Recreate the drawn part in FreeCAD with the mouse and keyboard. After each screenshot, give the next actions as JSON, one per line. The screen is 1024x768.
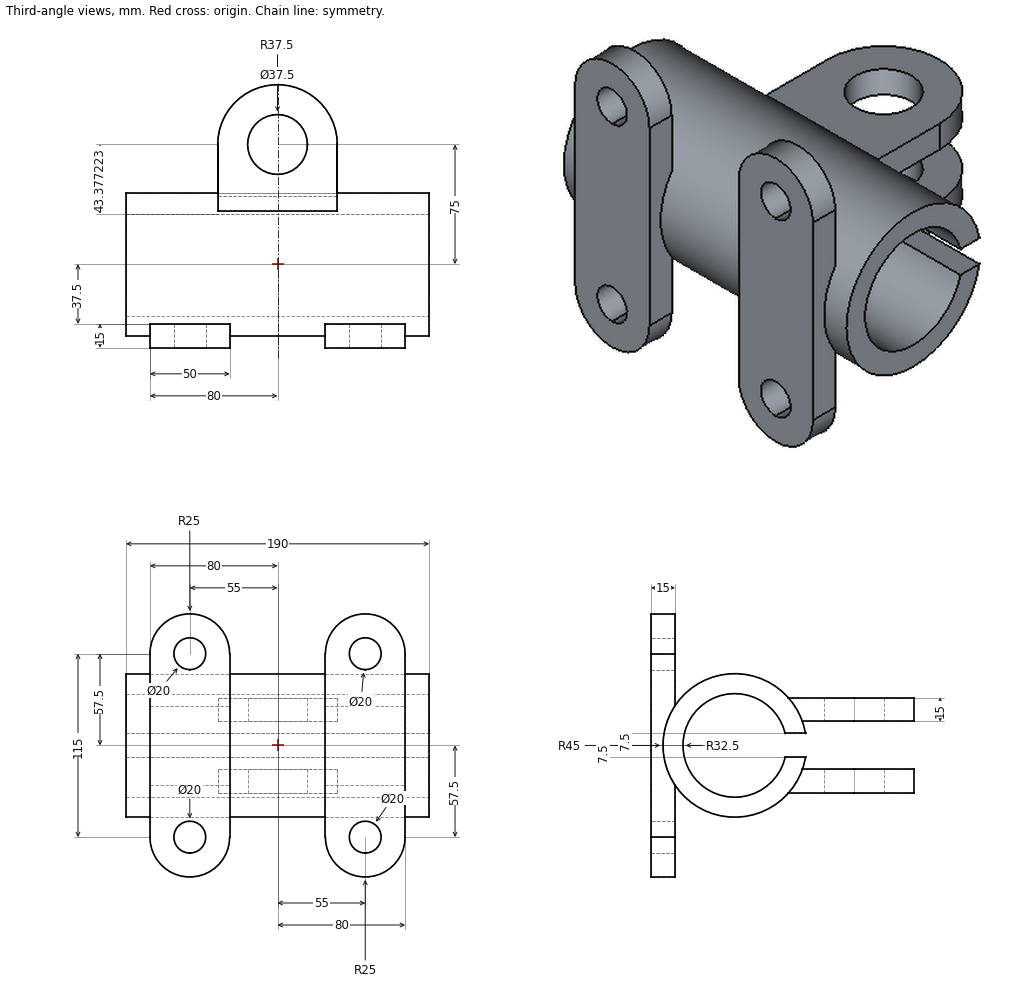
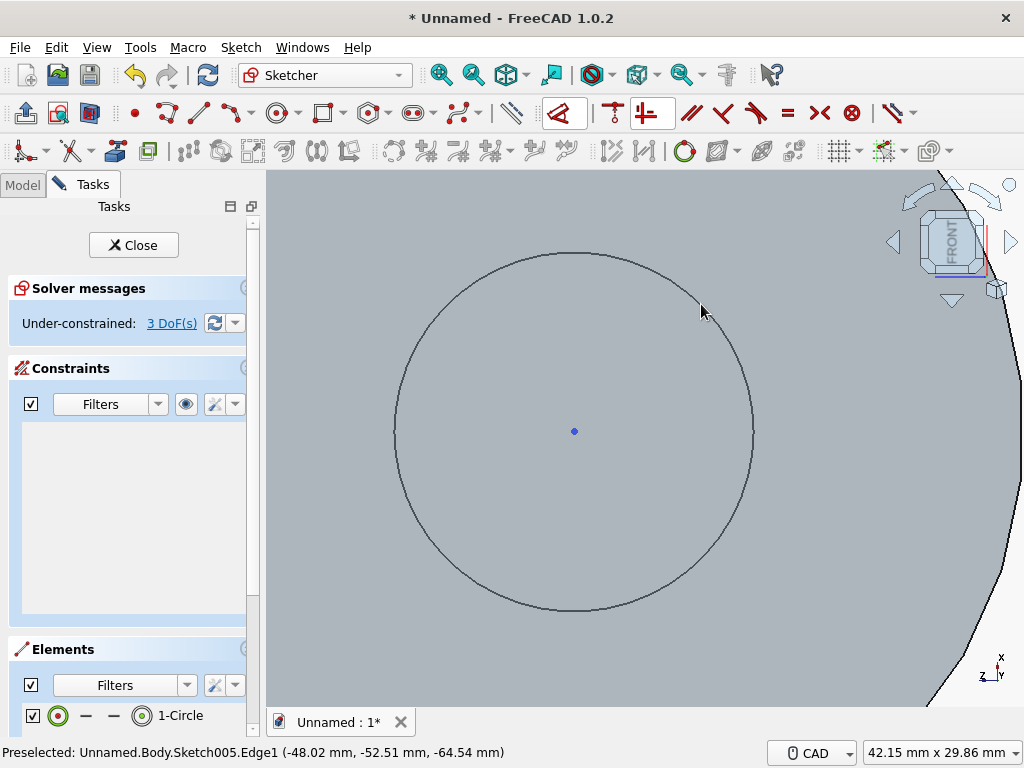
{"action": "left_click", "coordinate": [701, 305]}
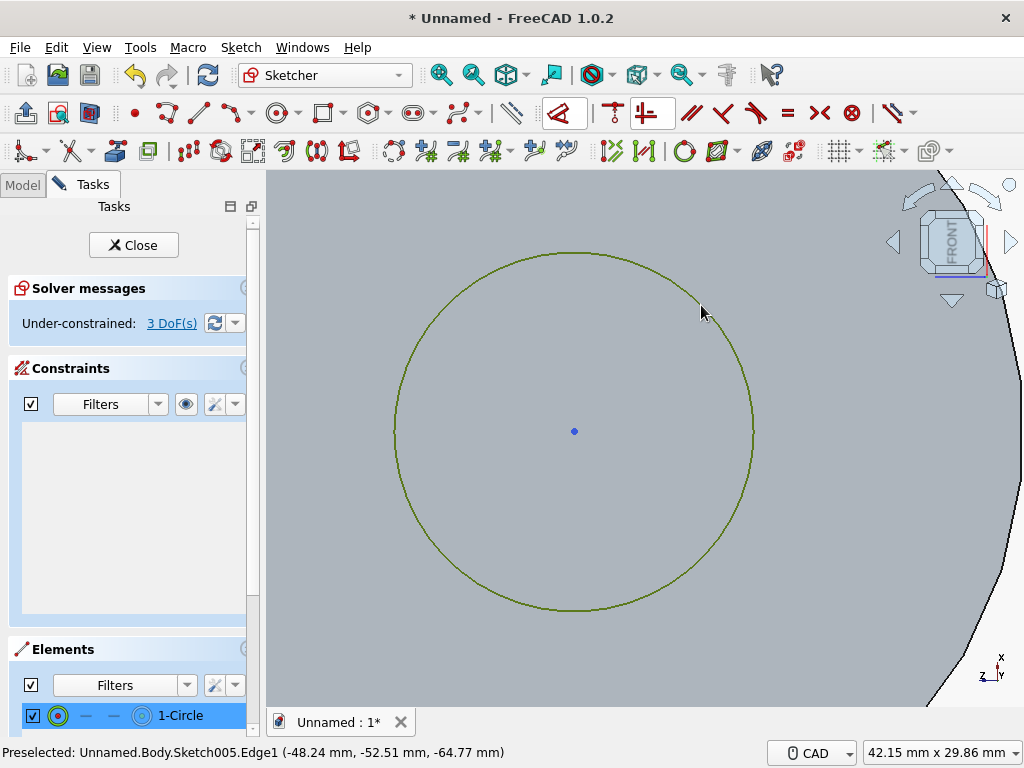
{"action": "left_click", "coordinate": [582, 114]}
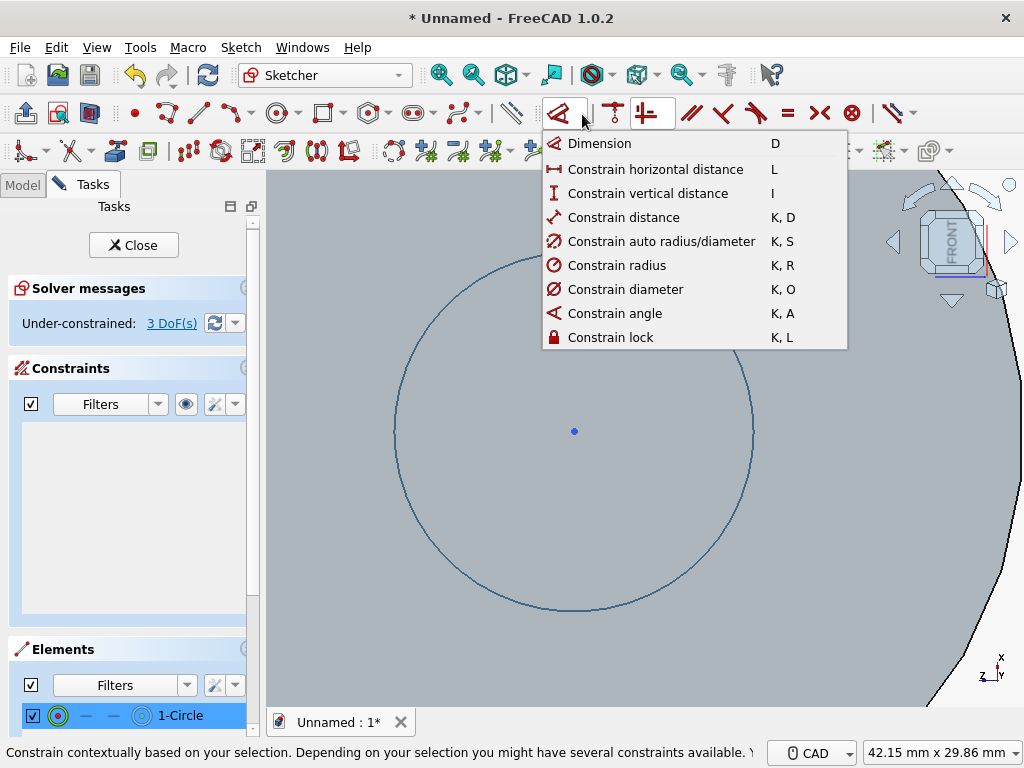
{"action": "left_click", "coordinate": [695, 289]}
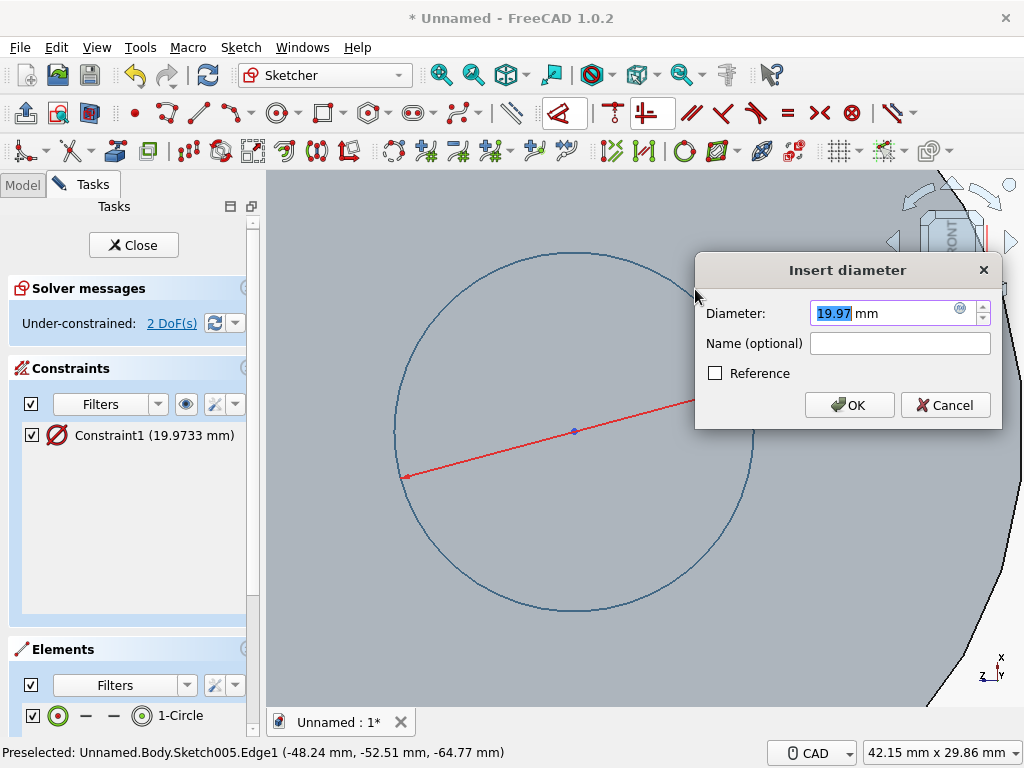
{"action": "type", "text": "20"}
{"action": "key", "text": "Return"}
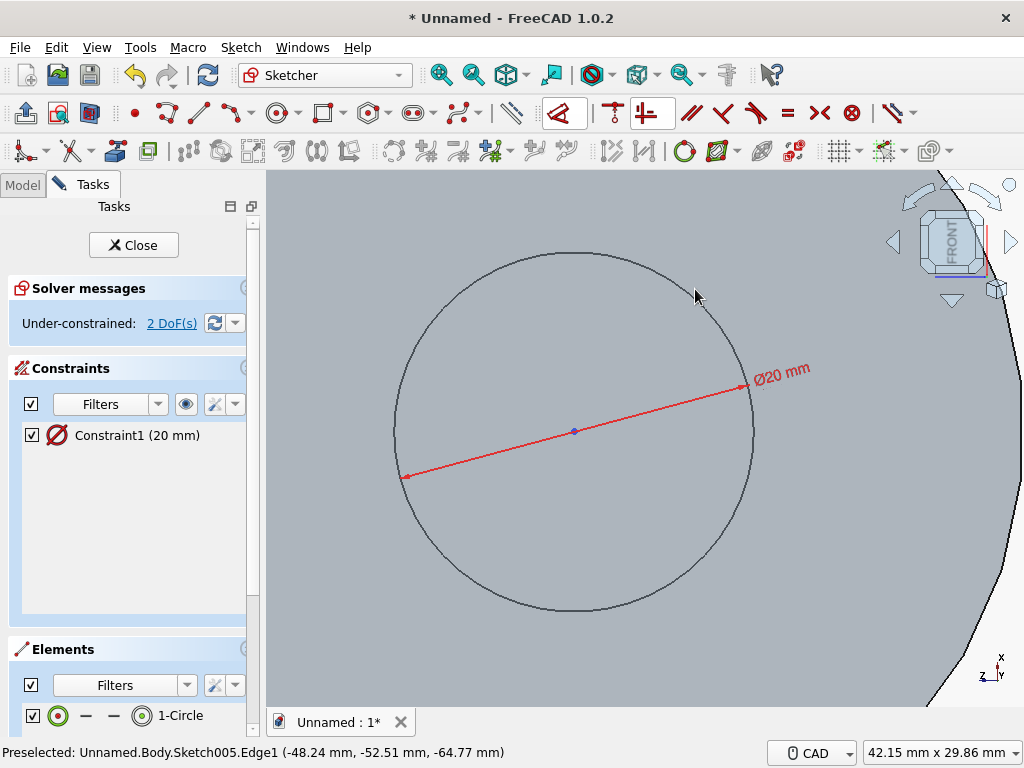
{"action": "left_click", "coordinate": [574, 432]}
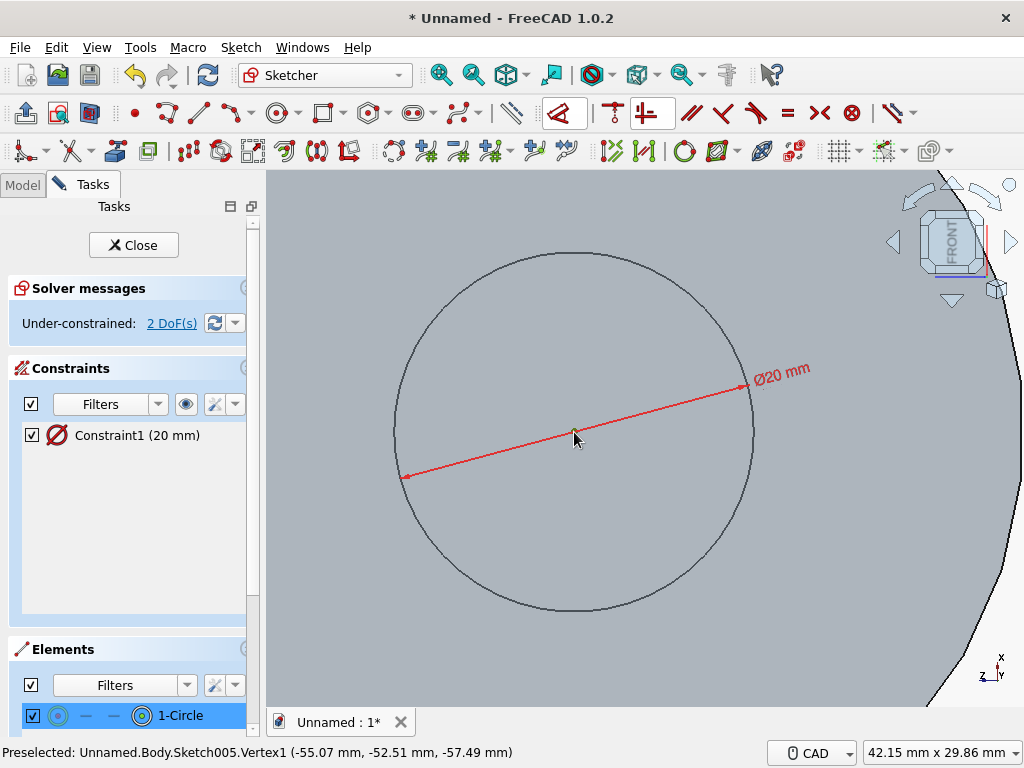
{"action": "left_click", "coordinate": [582, 114]}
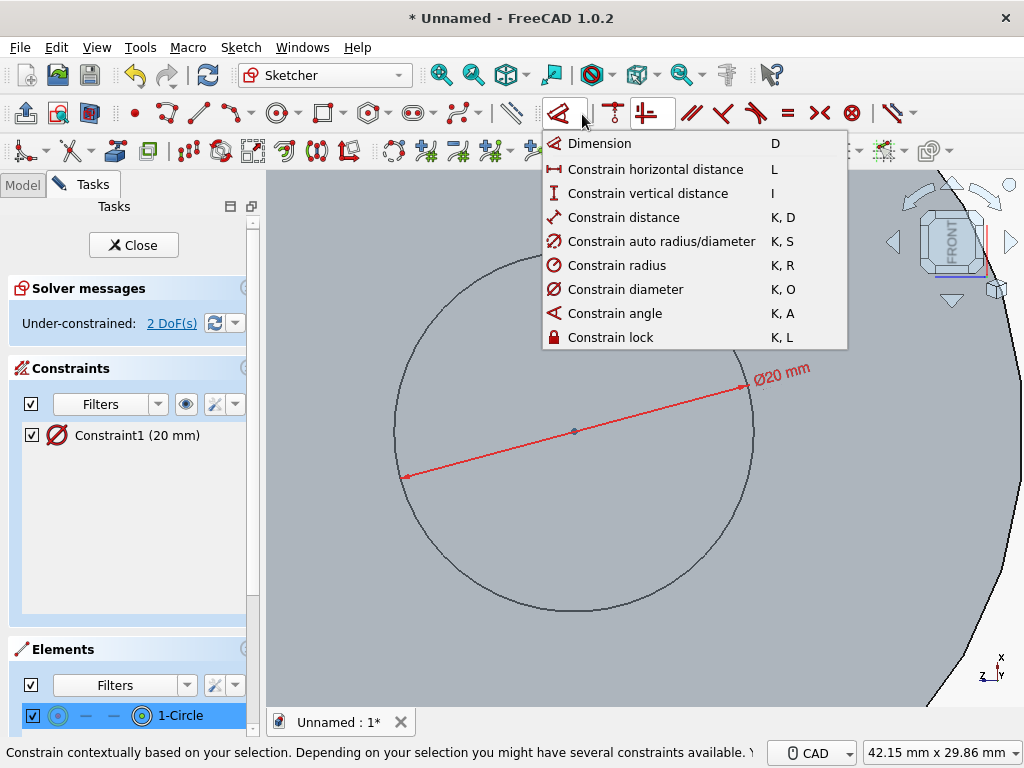
{"action": "left_click", "coordinate": [695, 193]}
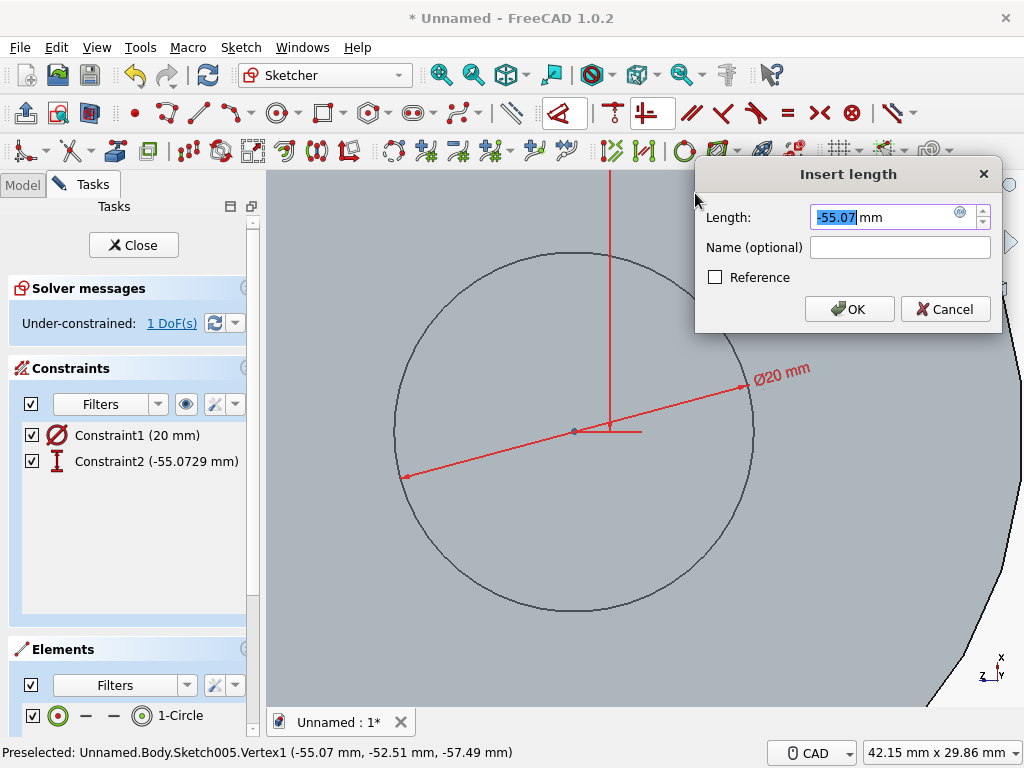
{"action": "type", "text": "-55"}
{"action": "key", "text": "Return"}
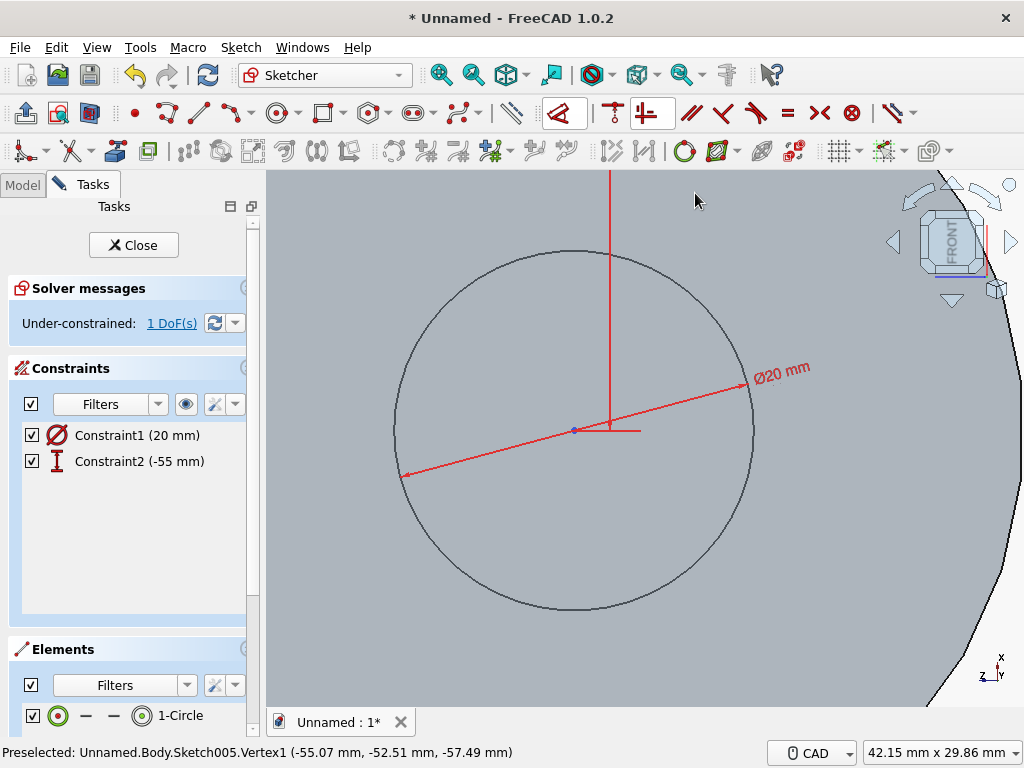
{"action": "left_click", "coordinate": [574, 431]}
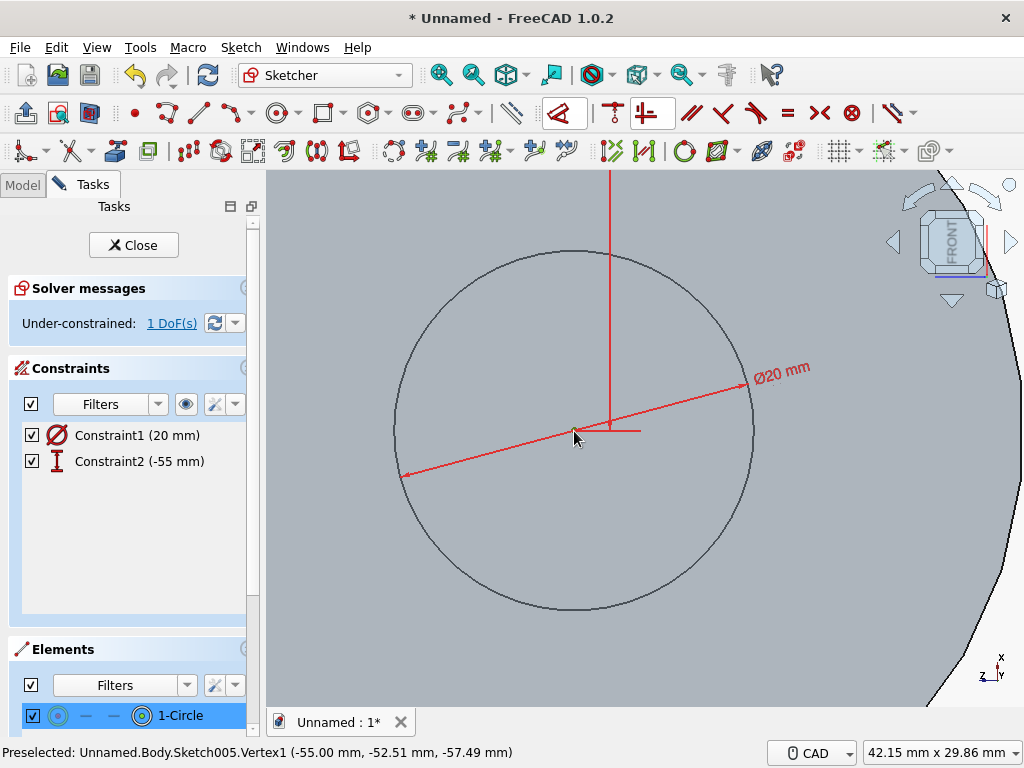
{"action": "key", "text": "l"}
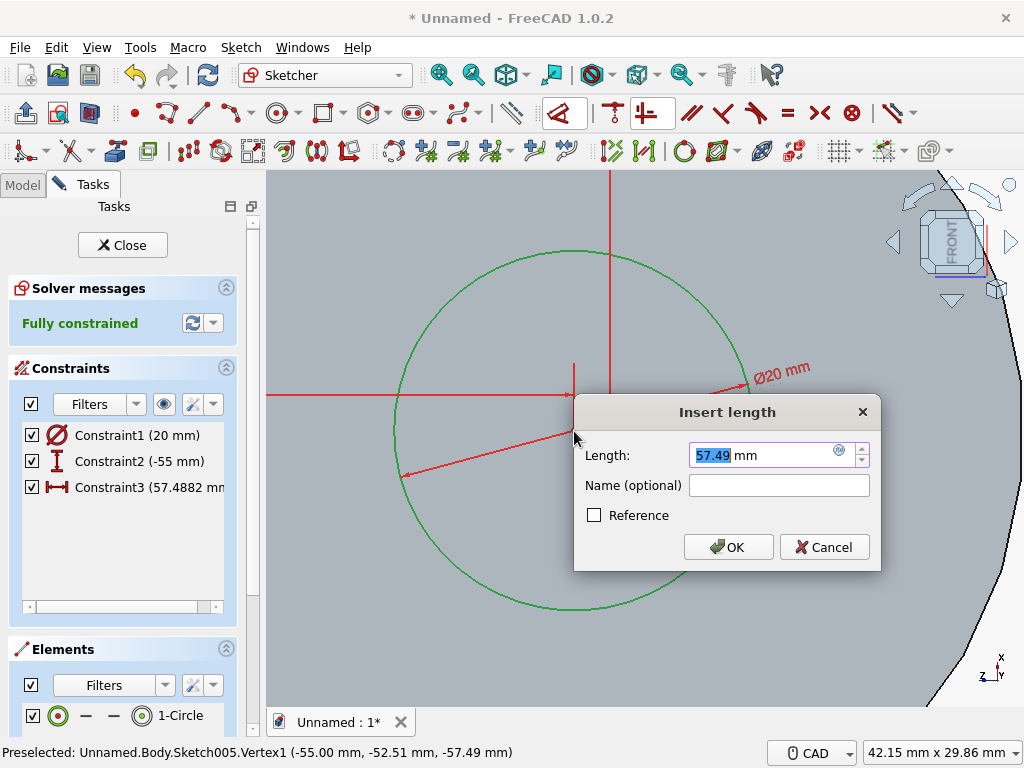
{"action": "type", "text": "57.5"}
{"action": "key", "text": "Return"}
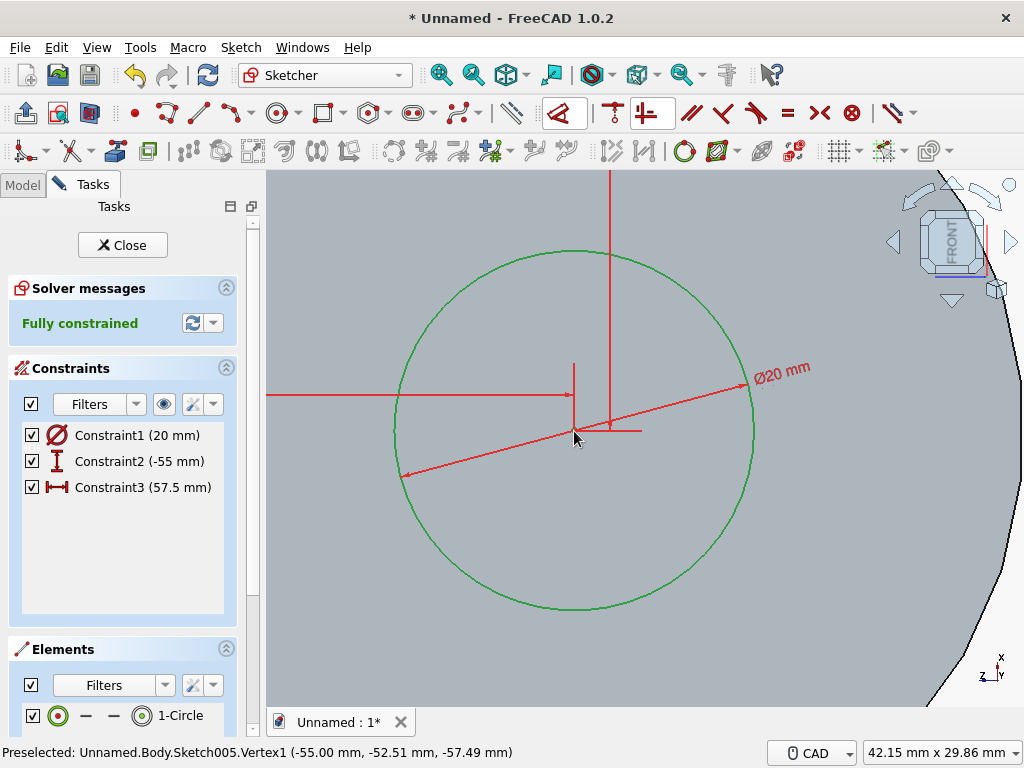
{"action": "left_click", "coordinate": [123, 245]}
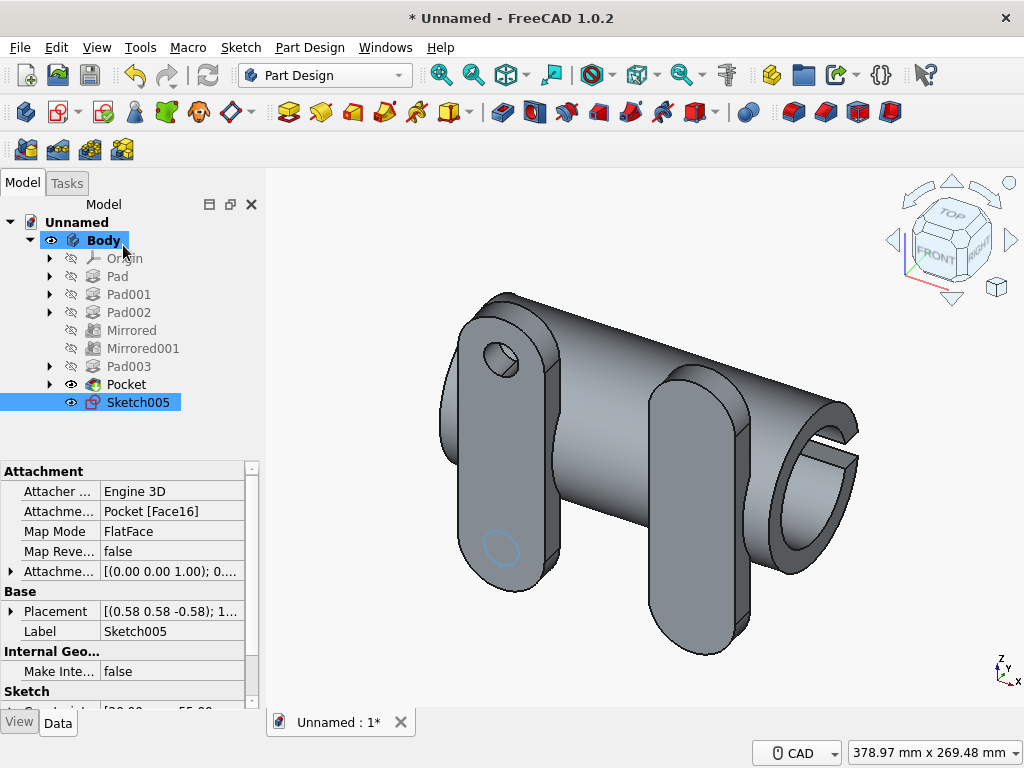
{"action": "left_click", "coordinate": [504, 112]}